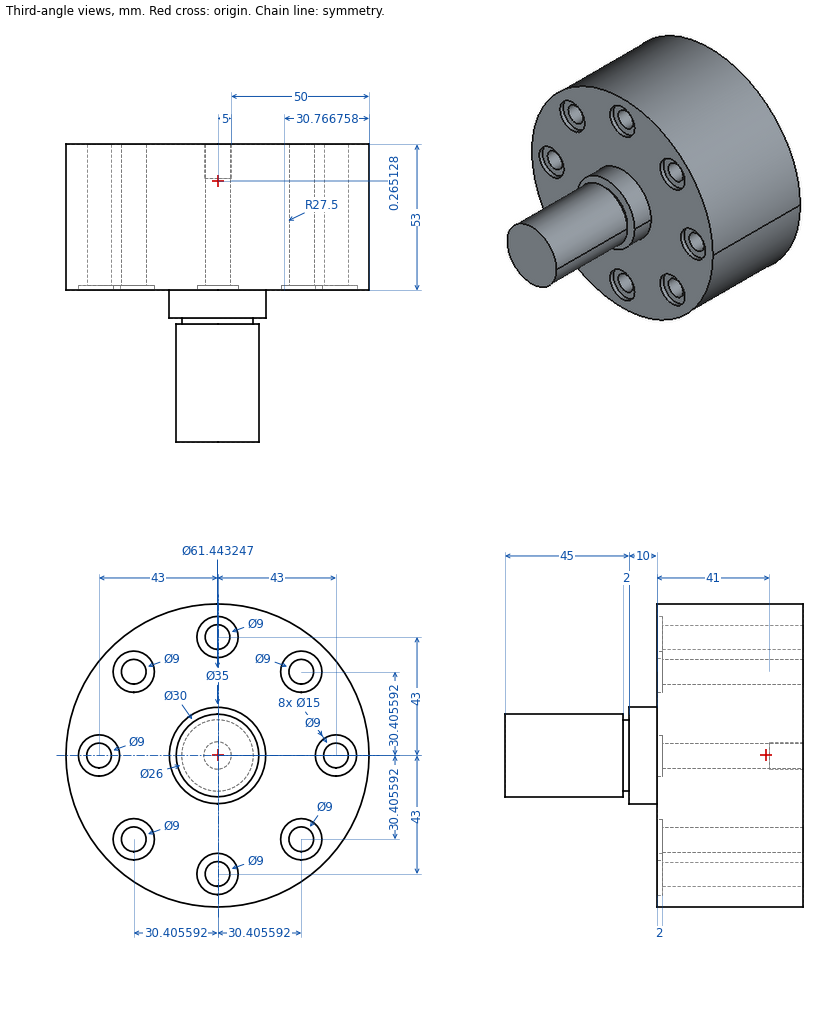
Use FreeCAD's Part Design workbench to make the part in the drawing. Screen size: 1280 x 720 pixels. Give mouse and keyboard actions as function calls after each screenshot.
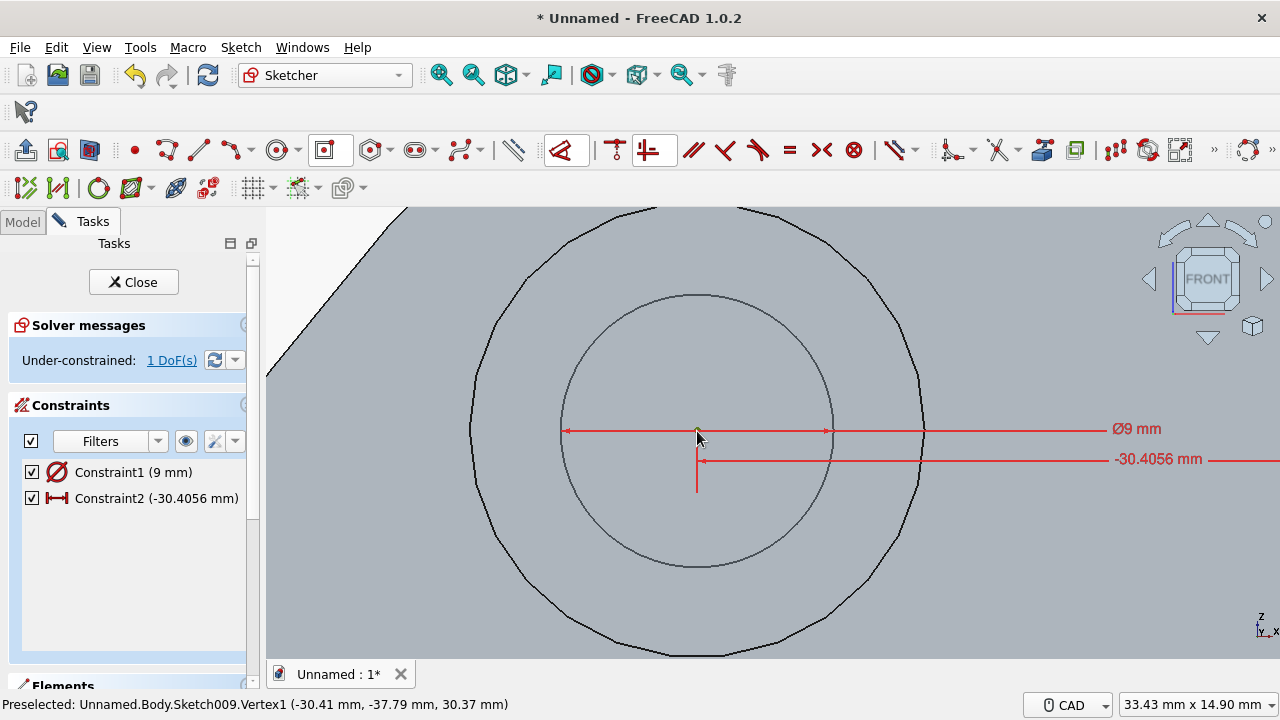
key(i)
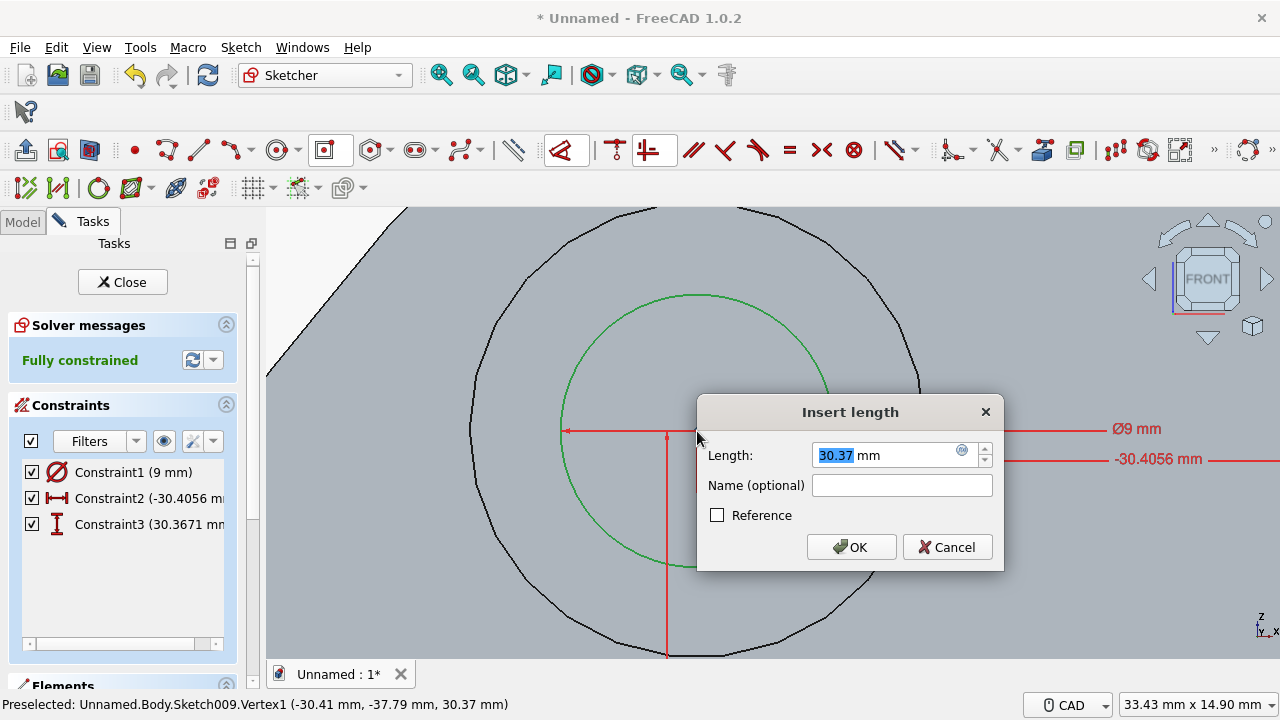
text(30.405592)
key(Return)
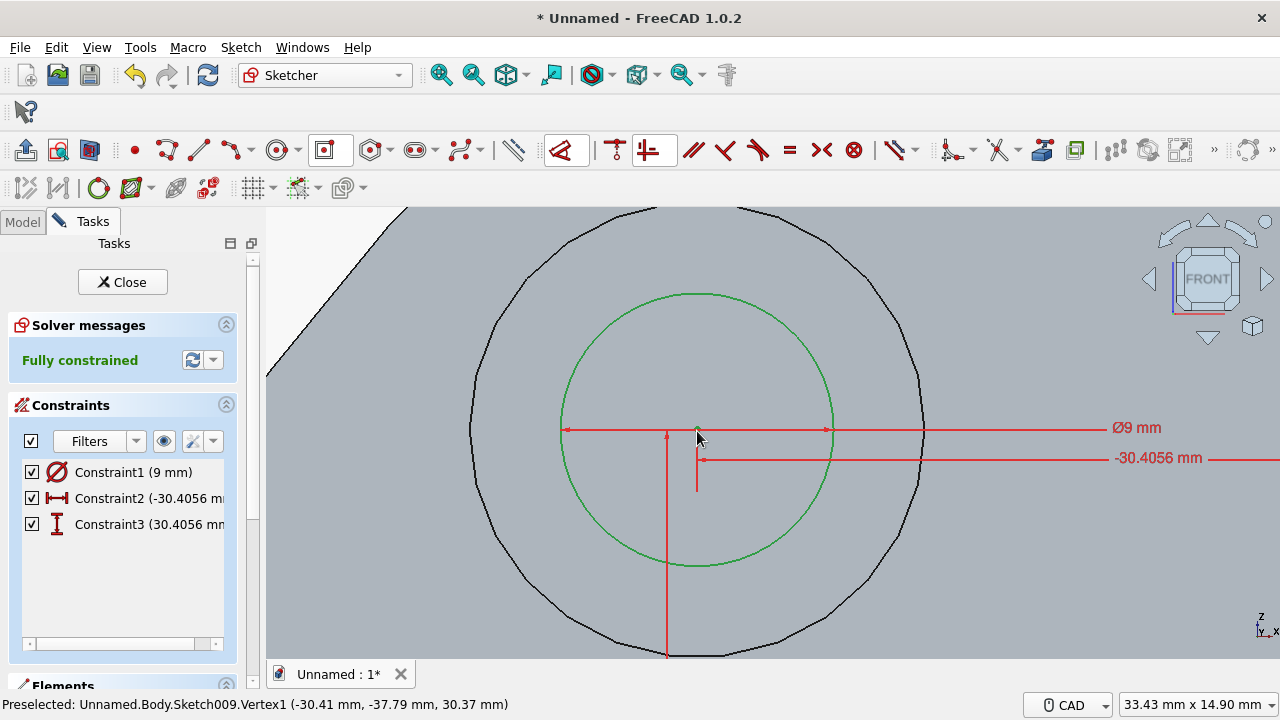
click(123, 282)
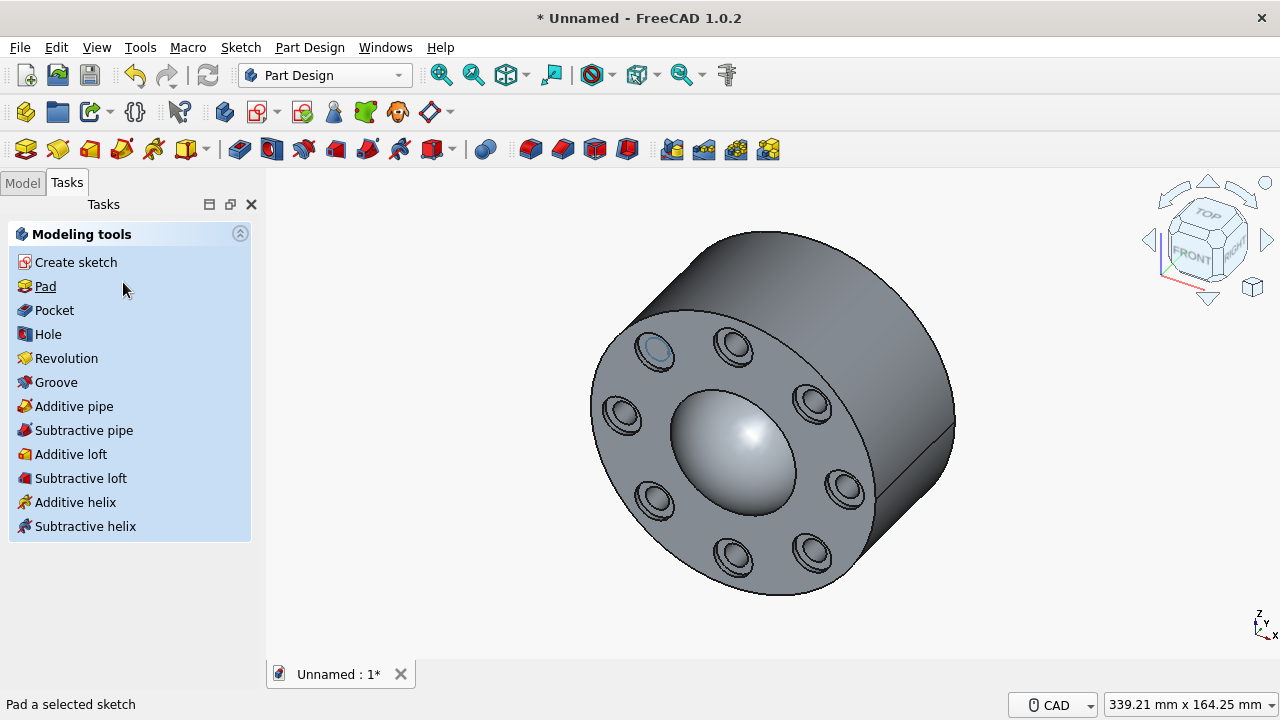
click(240, 150)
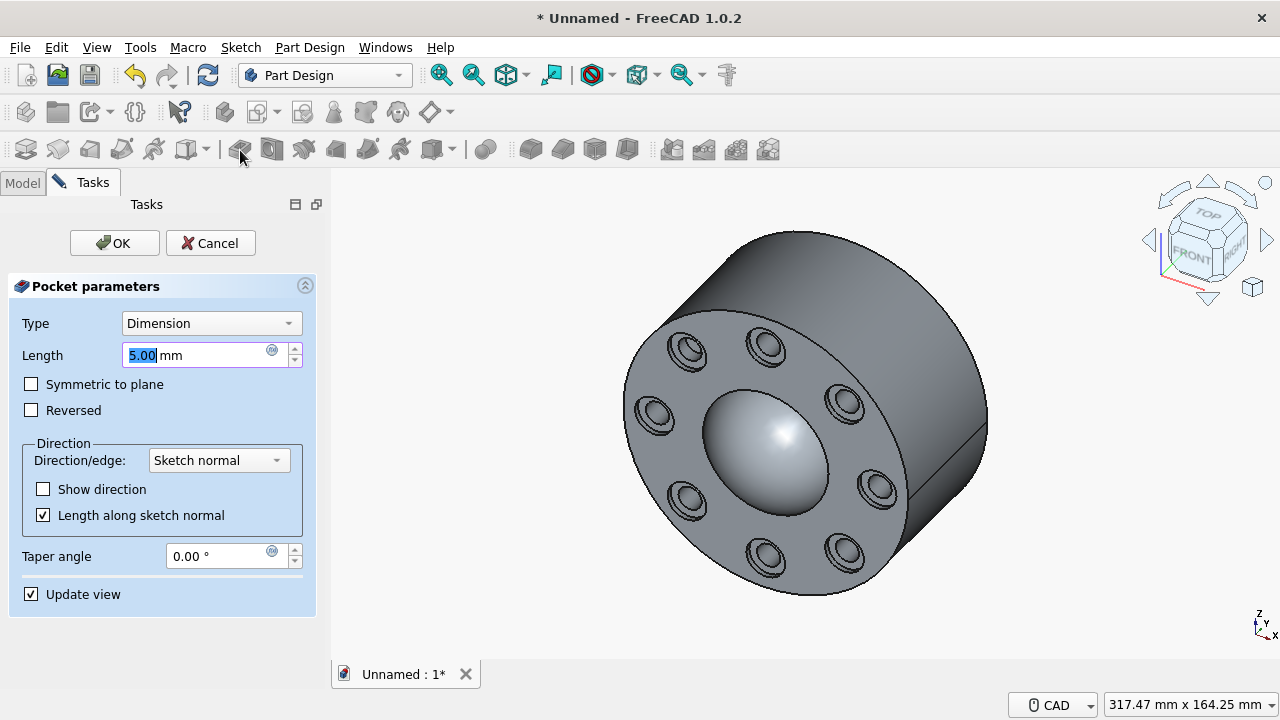
click(212, 324)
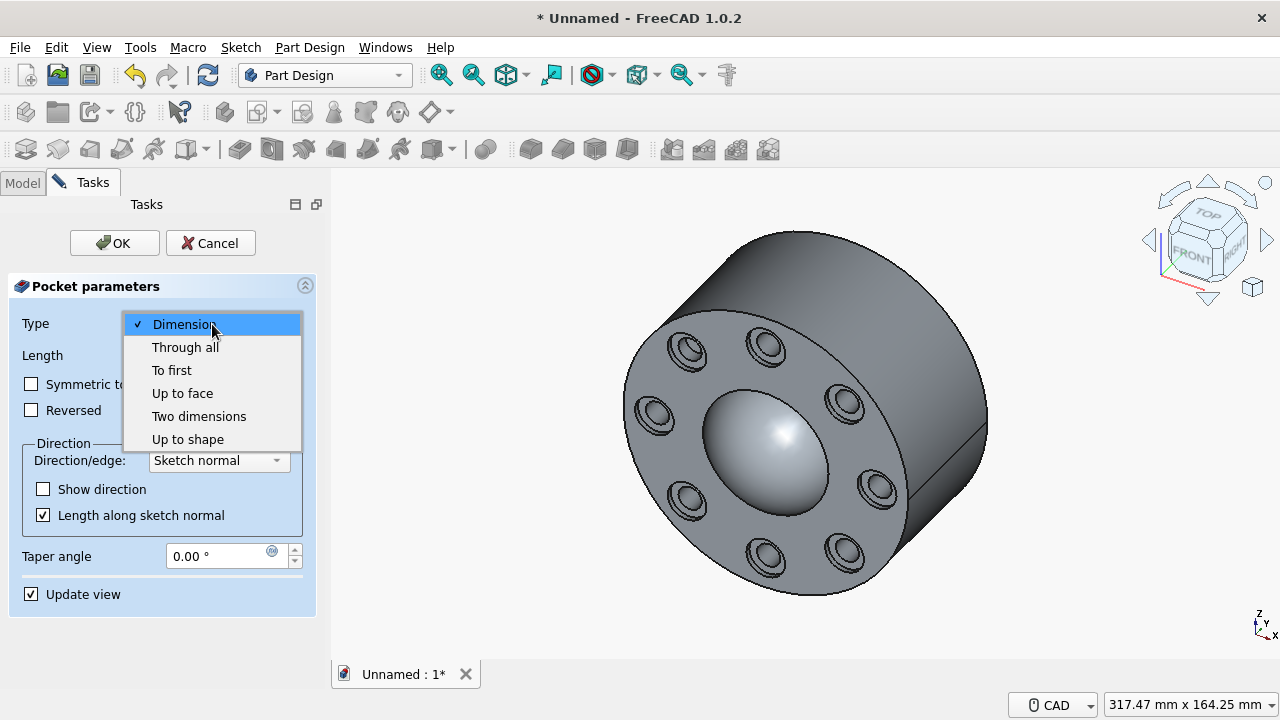
click(212, 370)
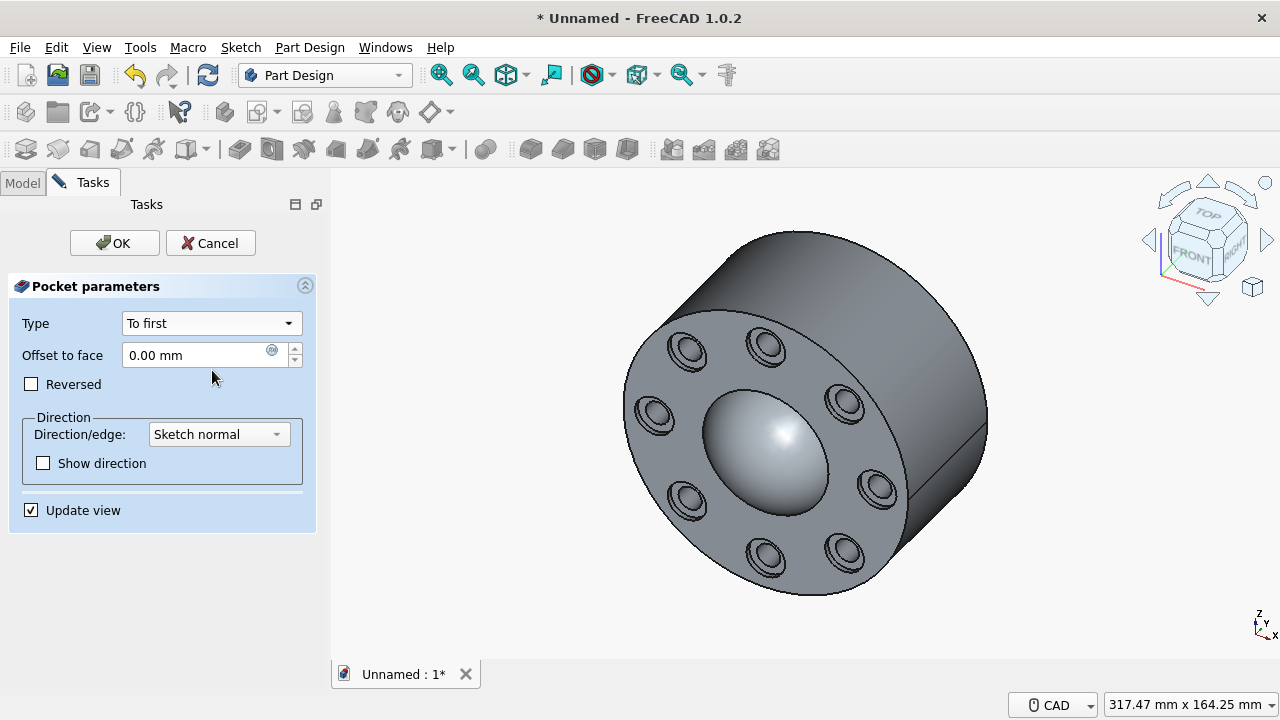
click(115, 243)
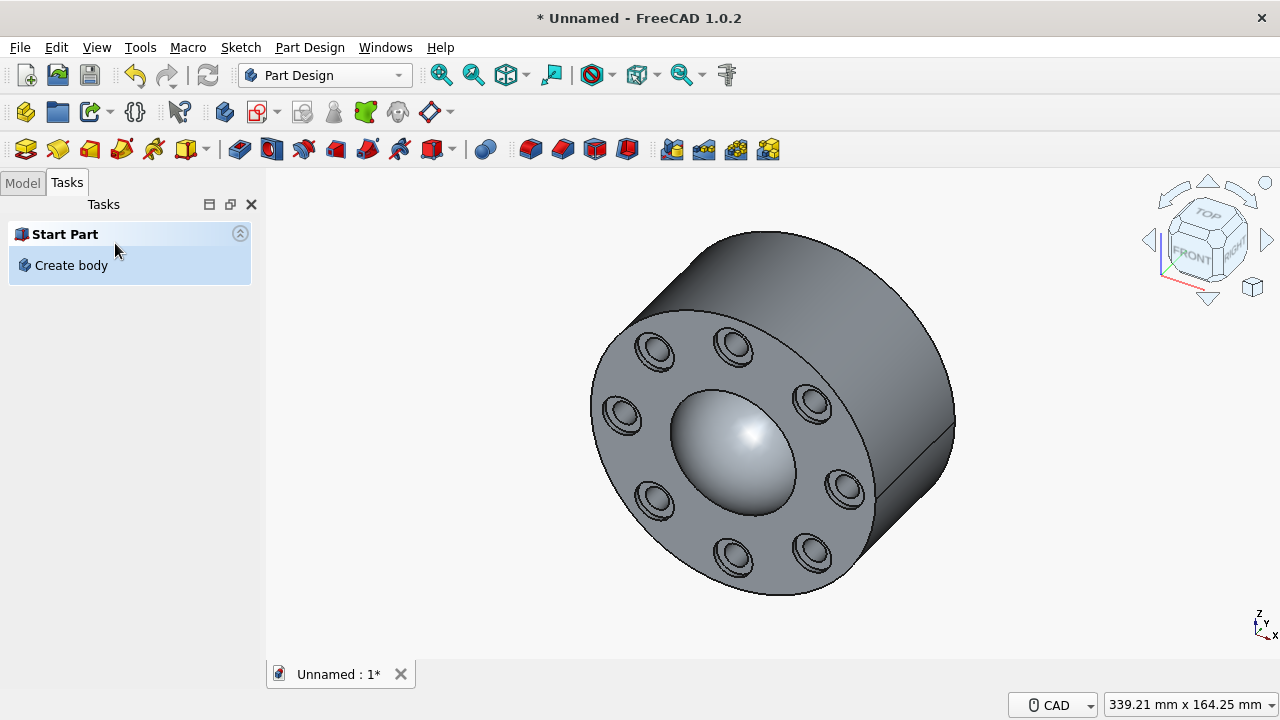
click(693, 361)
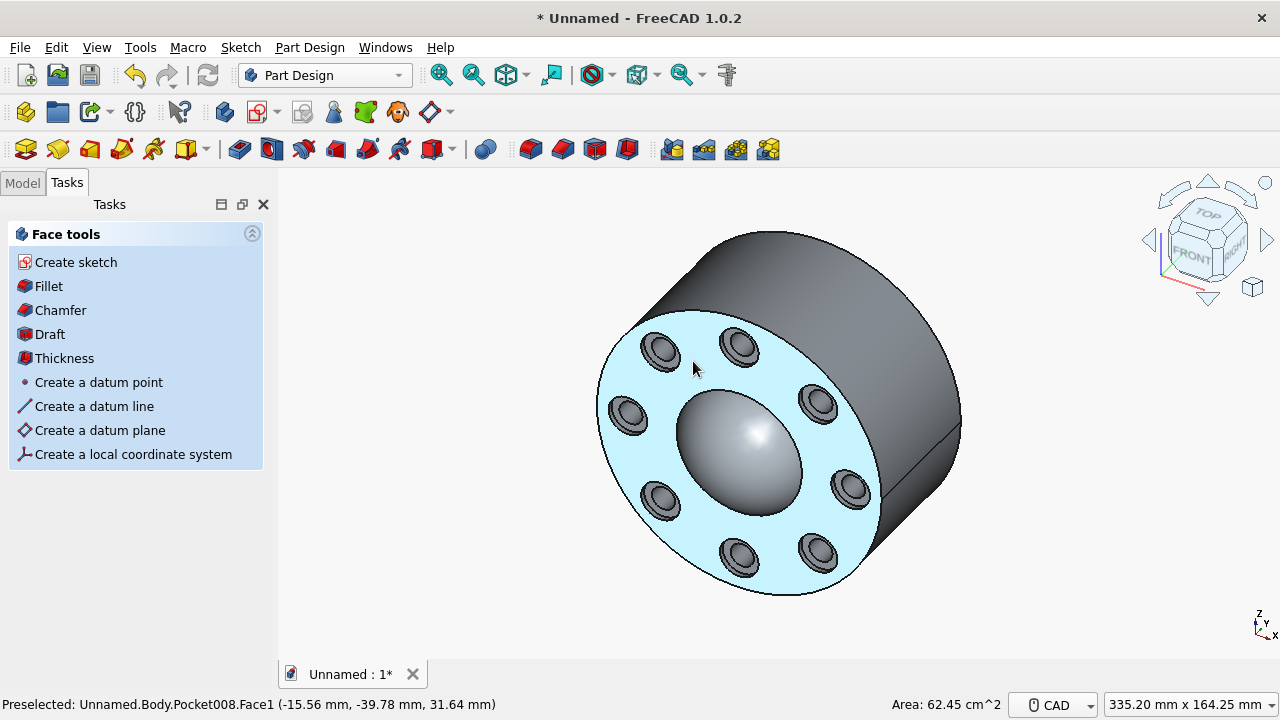
click(258, 112)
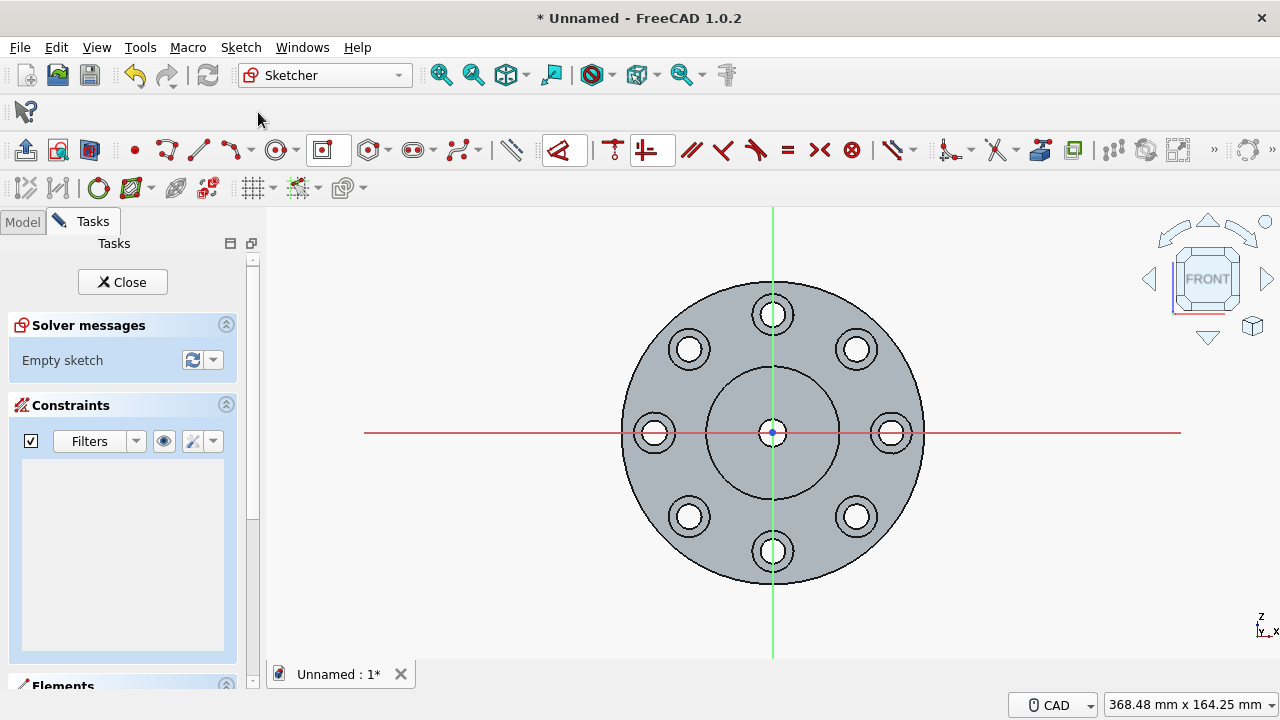
scroll(856, 433, up, 3)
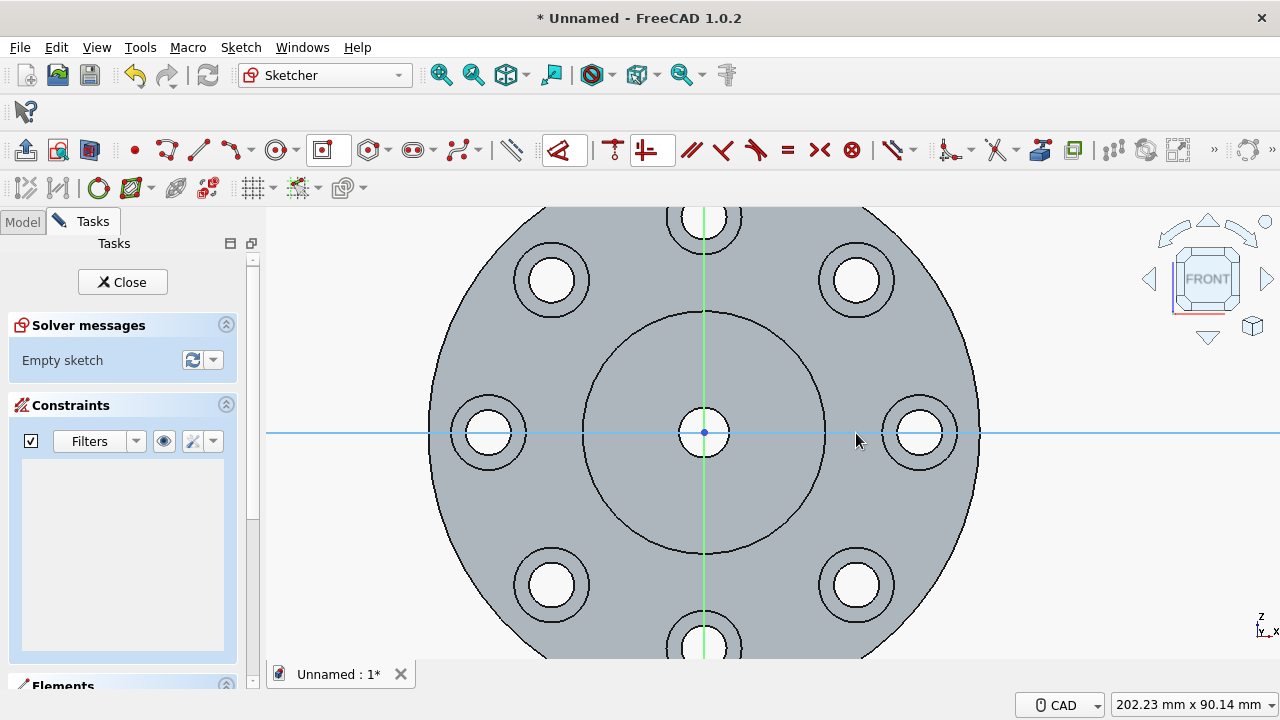
click(276, 150)